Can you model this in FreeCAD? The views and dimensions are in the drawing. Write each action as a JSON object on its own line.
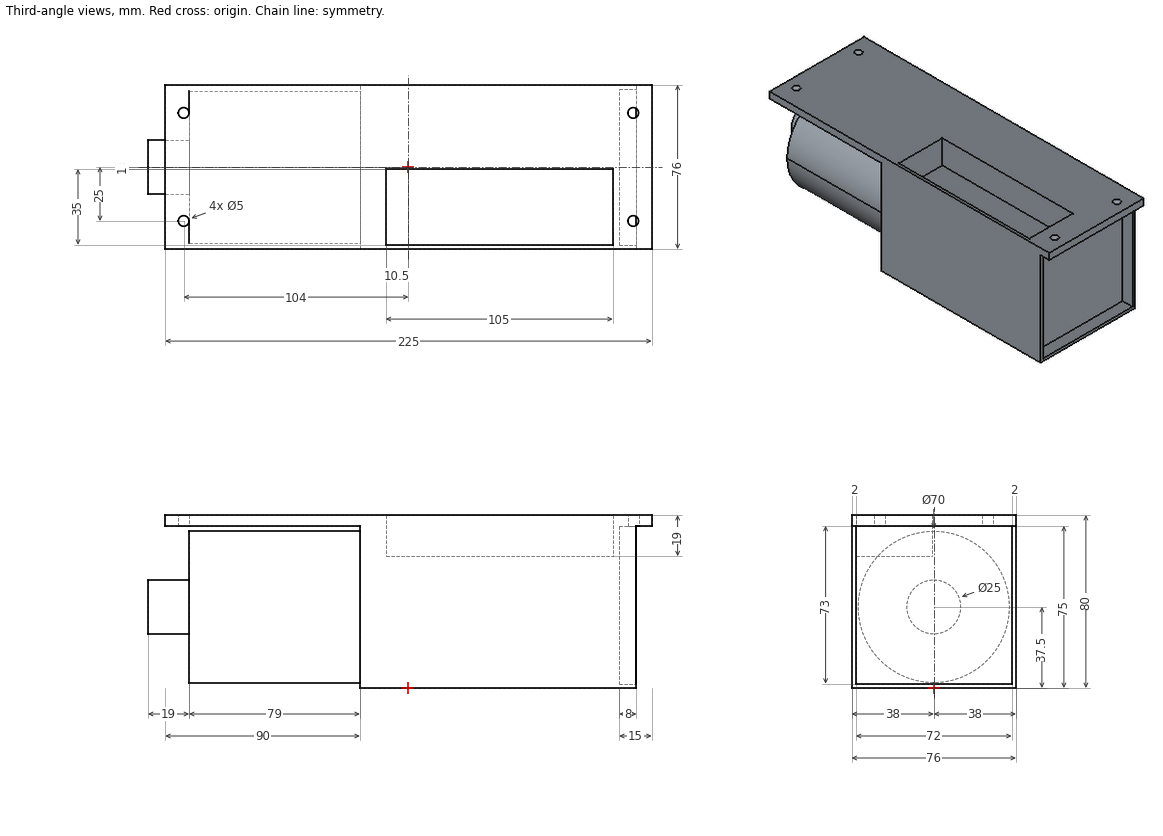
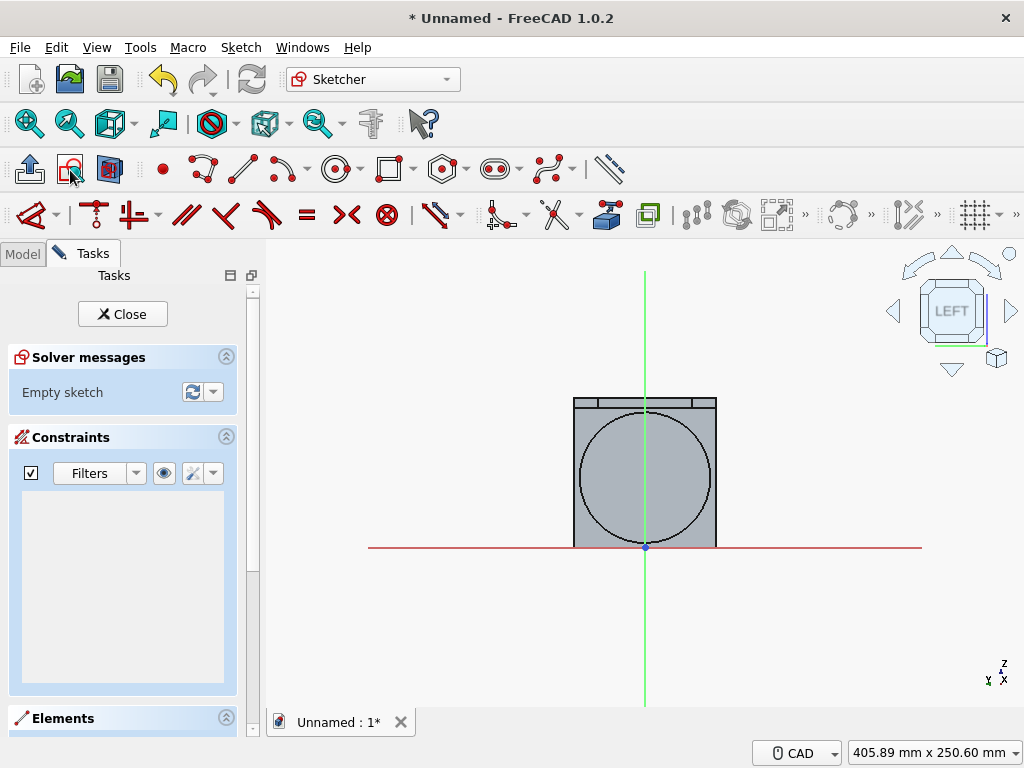
{"action": "scroll", "coordinate": [675, 513], "scroll_direction": "up", "scroll_amount": 6}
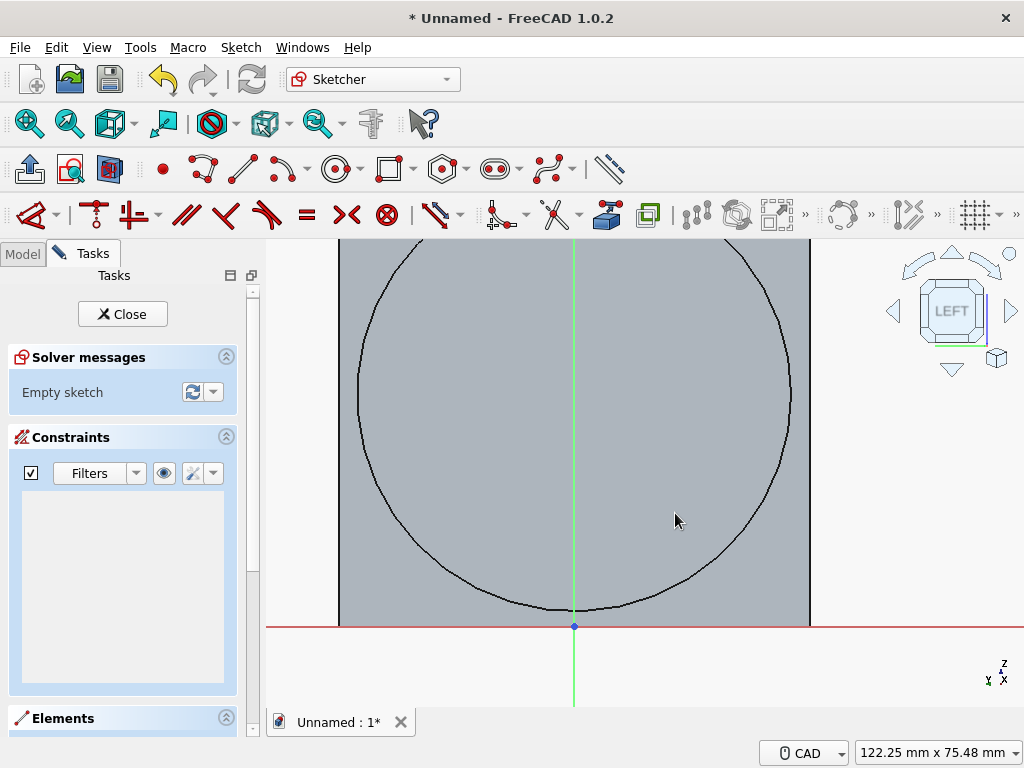
{"action": "key", "text": "g c"}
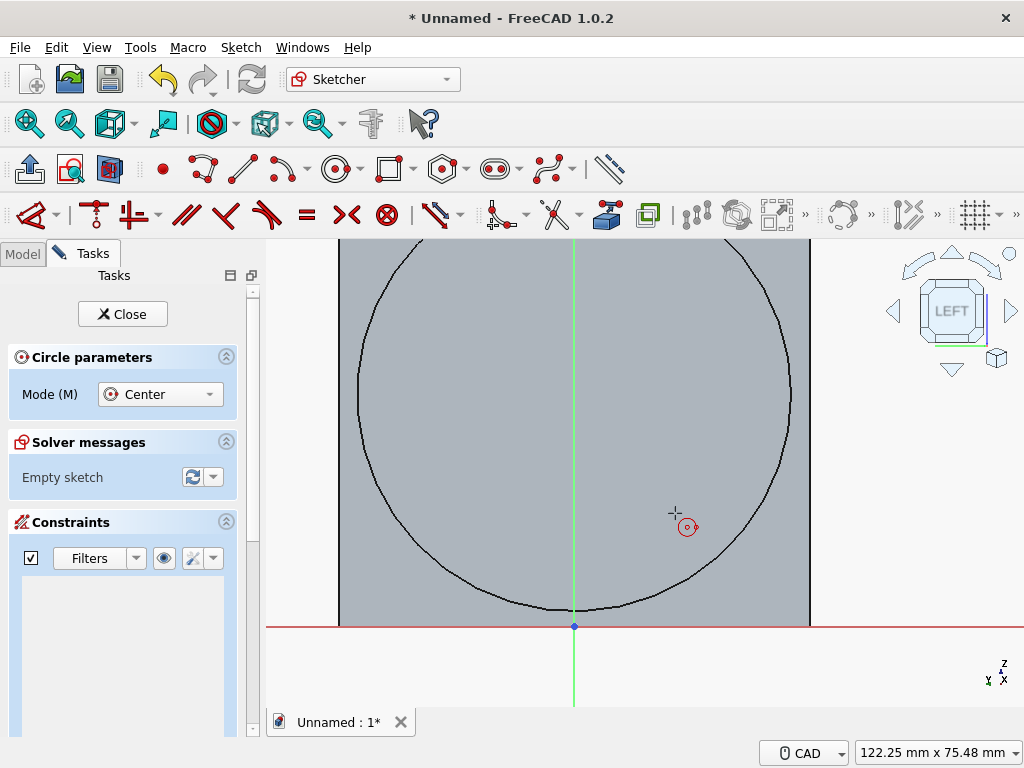
{"action": "left_click", "coordinate": [574, 394]}
{"action": "left_click", "coordinate": [629, 340]}
{"action": "key", "text": "Escape"}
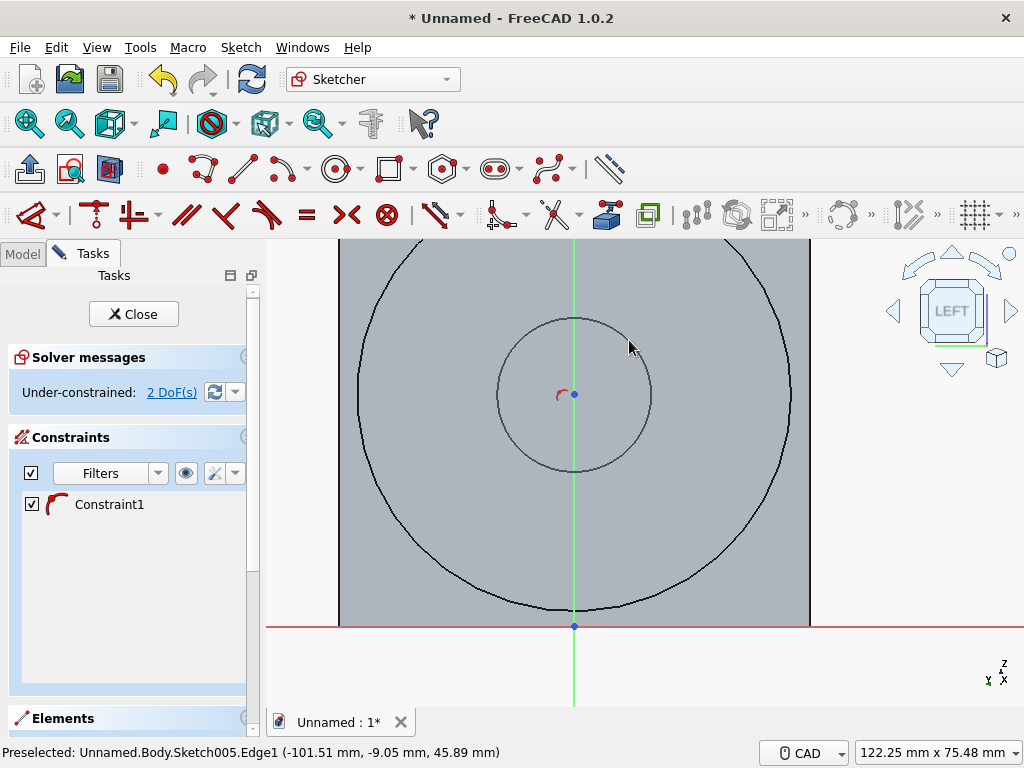
{"action": "left_click", "coordinate": [32, 216]}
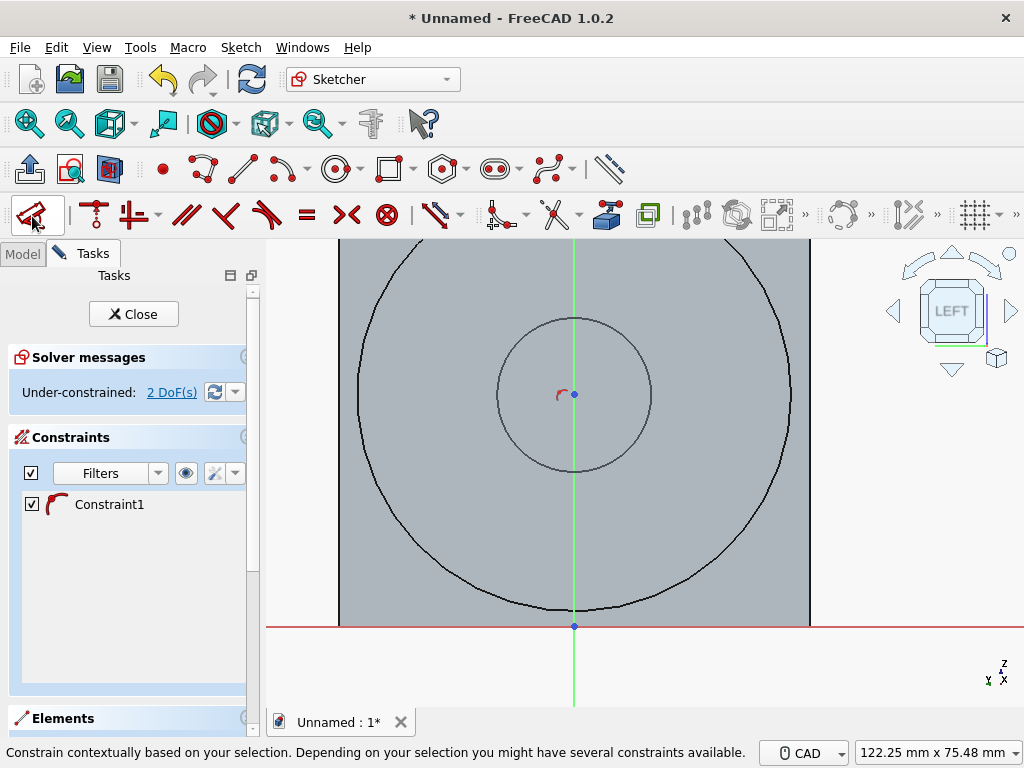
{"action": "left_click", "coordinate": [628, 340]}
{"action": "left_click", "coordinate": [650, 317]}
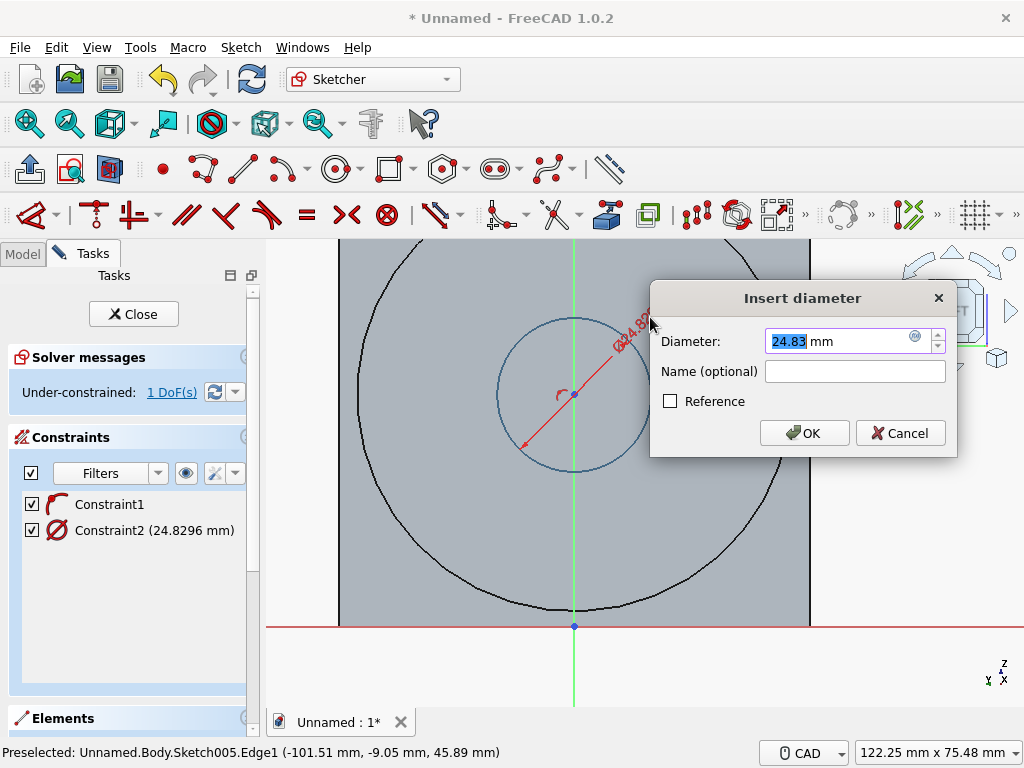
{"action": "type", "text": "25"}
{"action": "key", "text": "Return"}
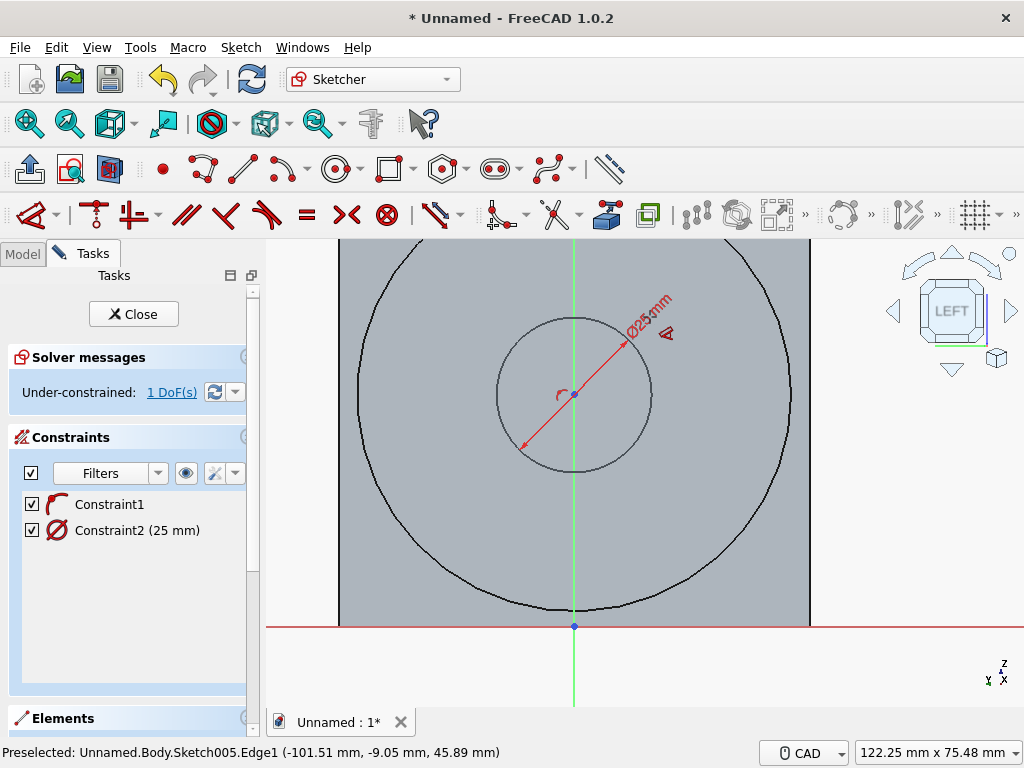
{"action": "left_click", "coordinate": [574, 395]}
{"action": "left_click", "coordinate": [608, 511]}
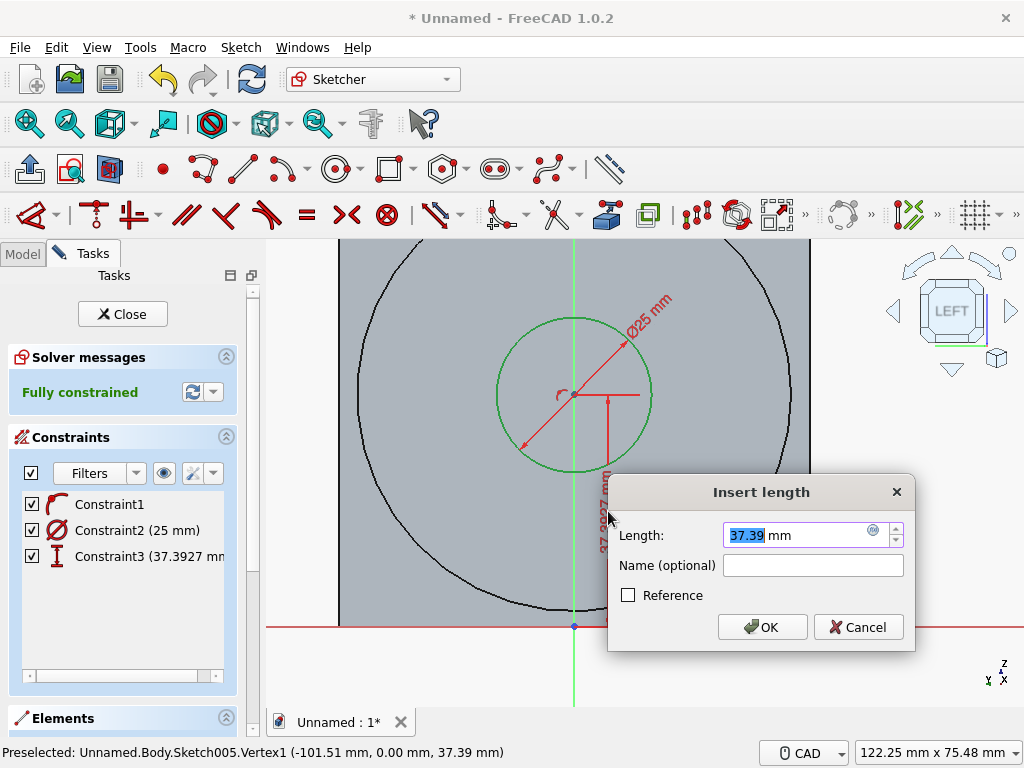
{"action": "type", "text": "37.5"}
{"action": "key", "text": "Return"}
{"action": "key", "text": "Escape"}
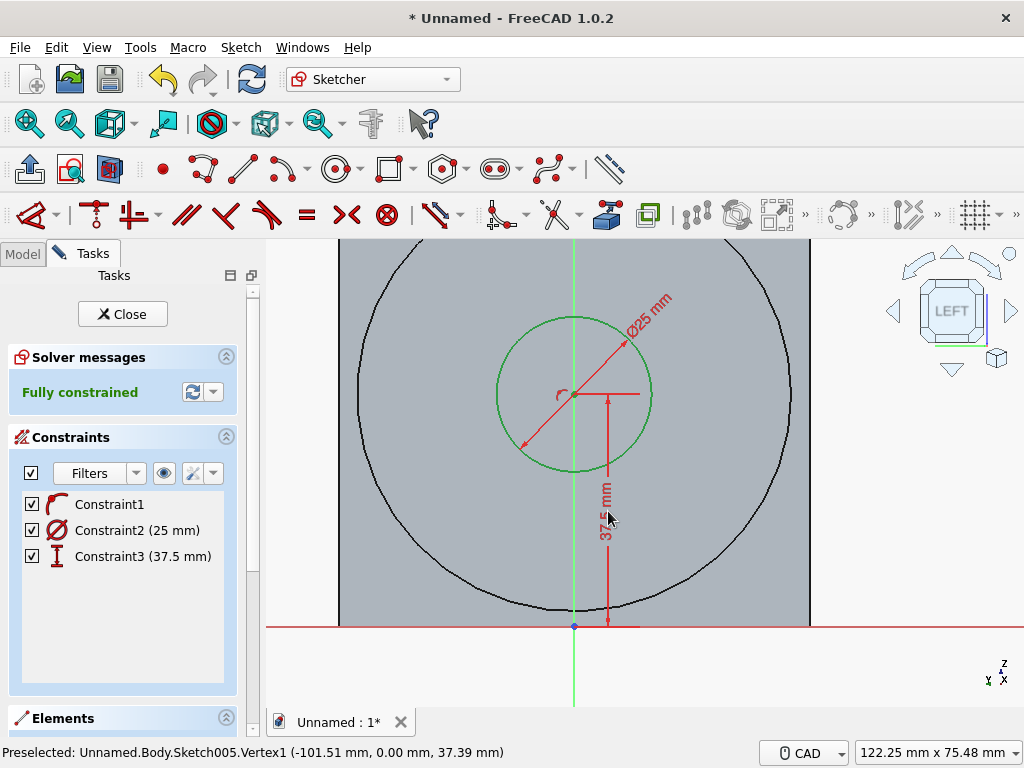
{"action": "left_click", "coordinate": [123, 314]}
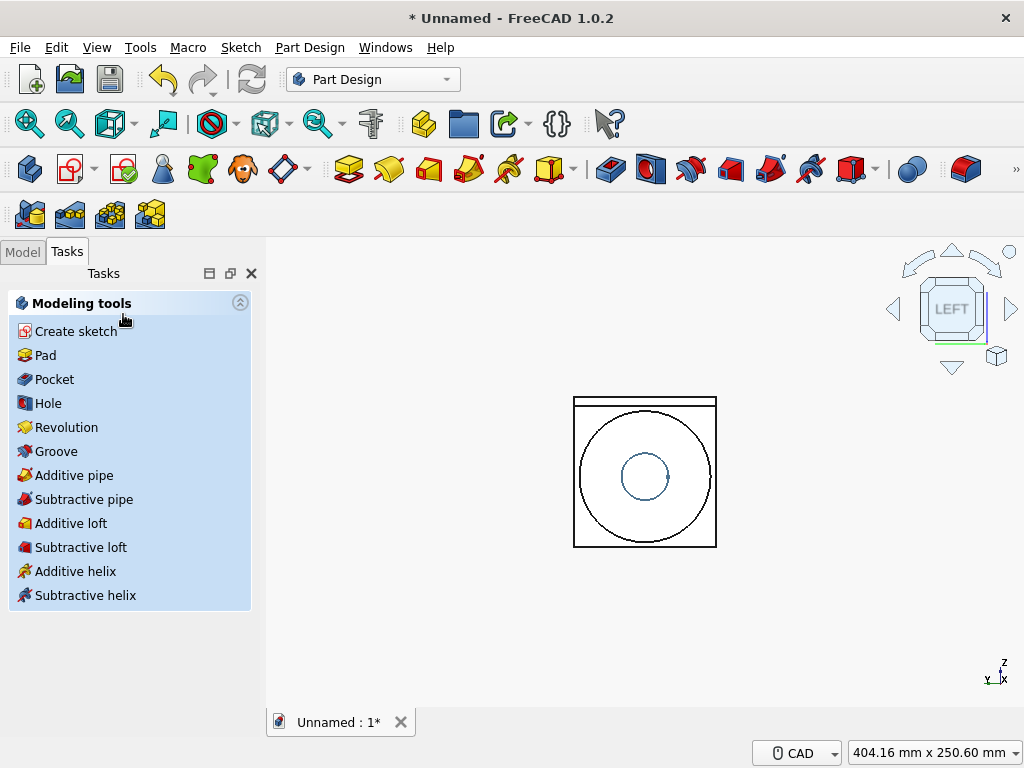
{"action": "left_click", "coordinate": [350, 170]}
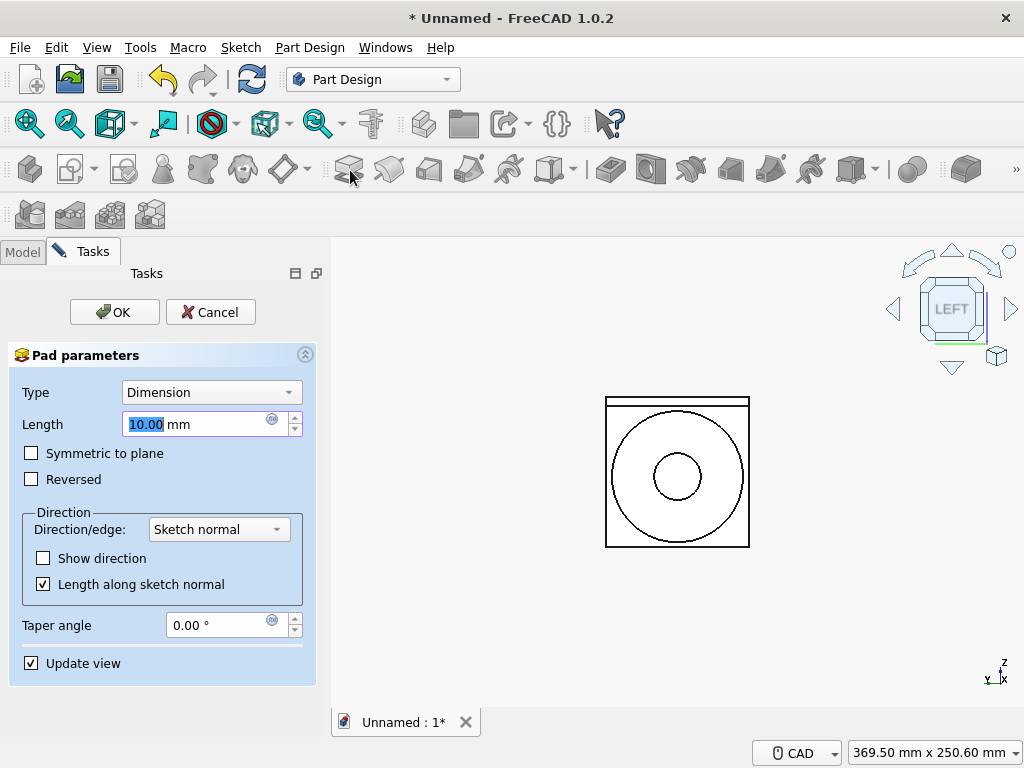
{"action": "type", "text": "19"}
{"action": "key", "text": "Tab"}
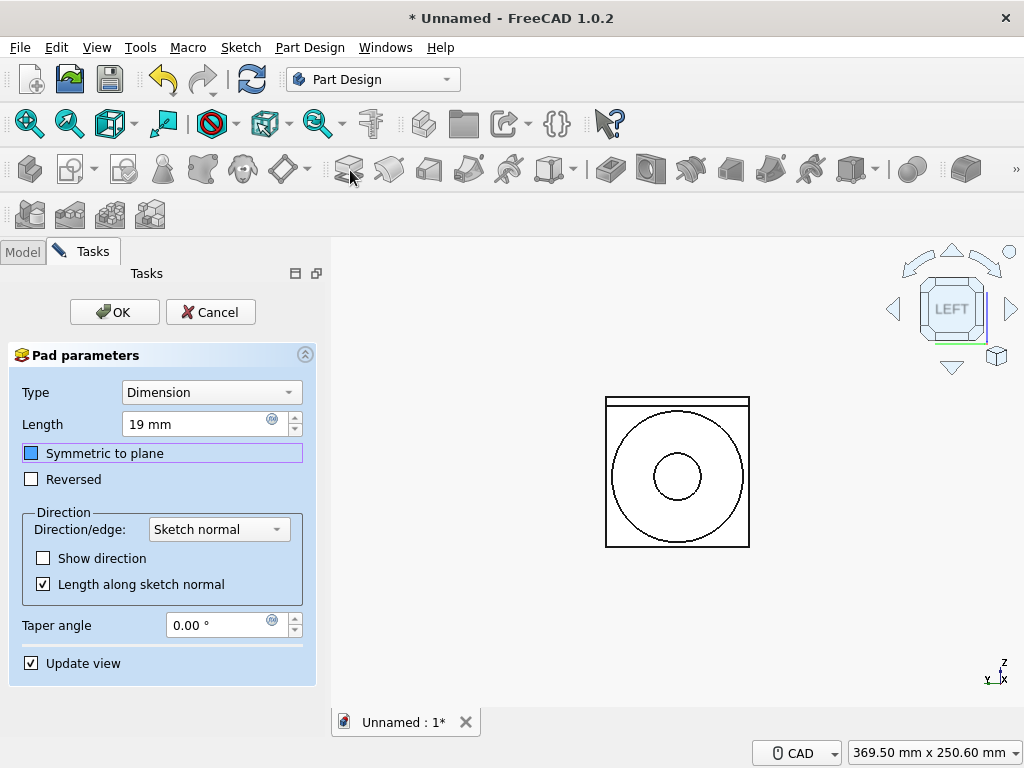
{"action": "left_click", "coordinate": [115, 312]}